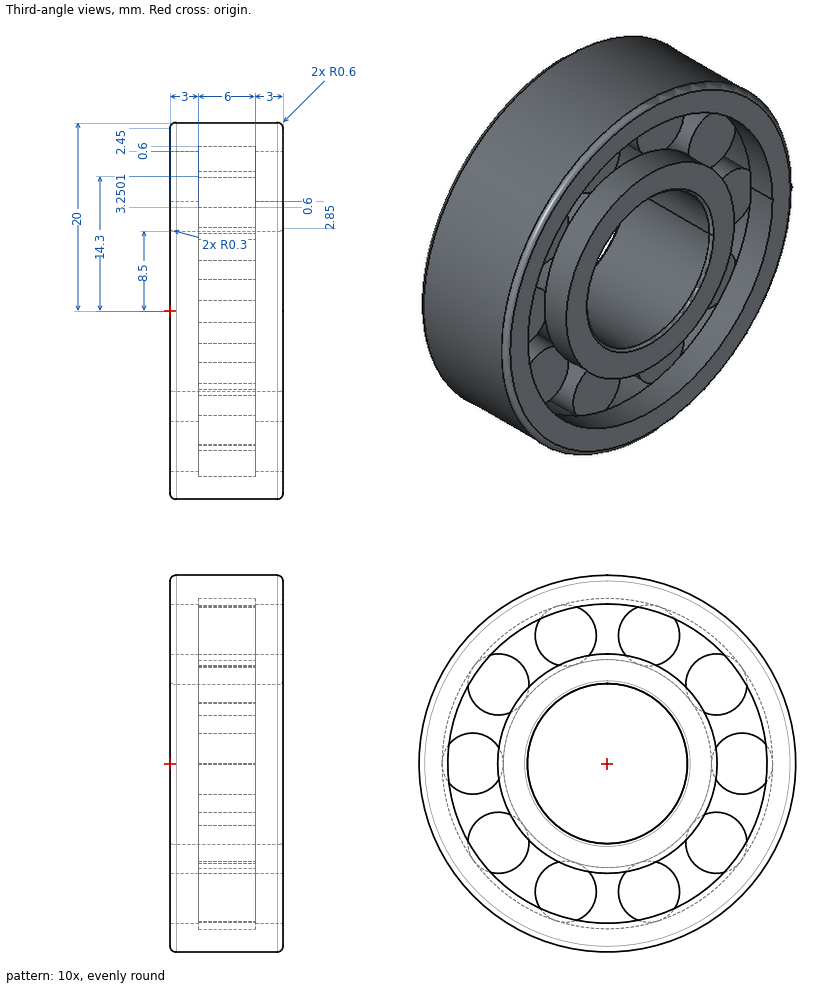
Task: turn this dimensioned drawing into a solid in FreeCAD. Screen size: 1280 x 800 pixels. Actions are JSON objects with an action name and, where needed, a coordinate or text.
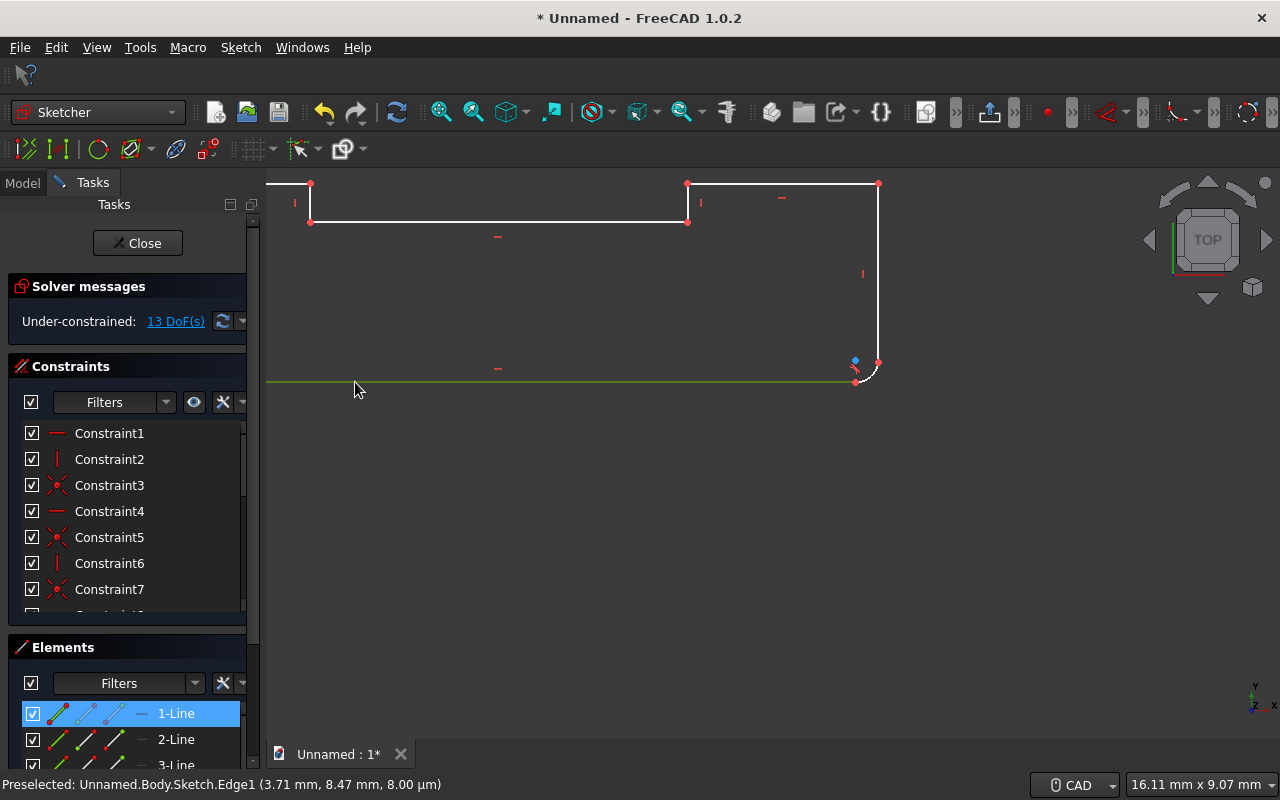
{"action": "scroll", "coordinate": [872, 376], "scroll_direction": "down", "scroll_amount": 4}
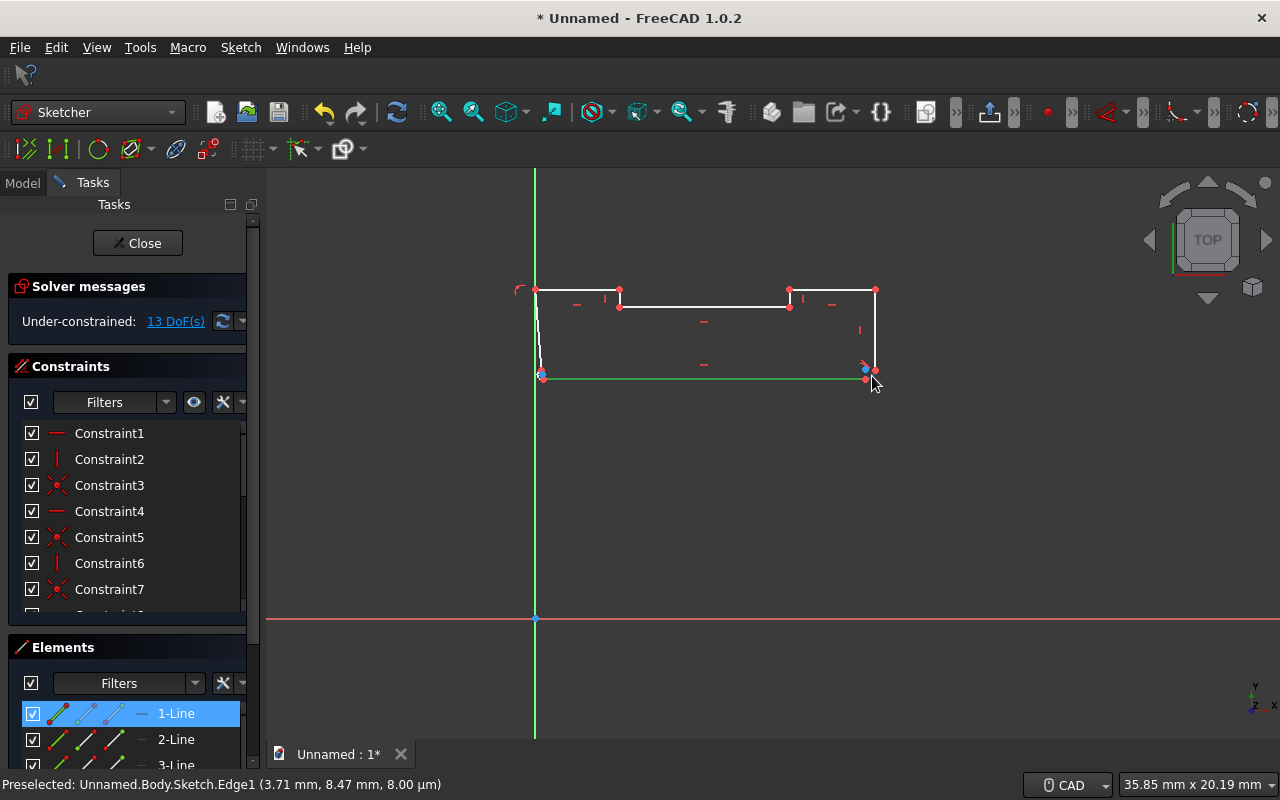
{"action": "scroll", "coordinate": [539, 378], "scroll_direction": "up", "scroll_amount": 7}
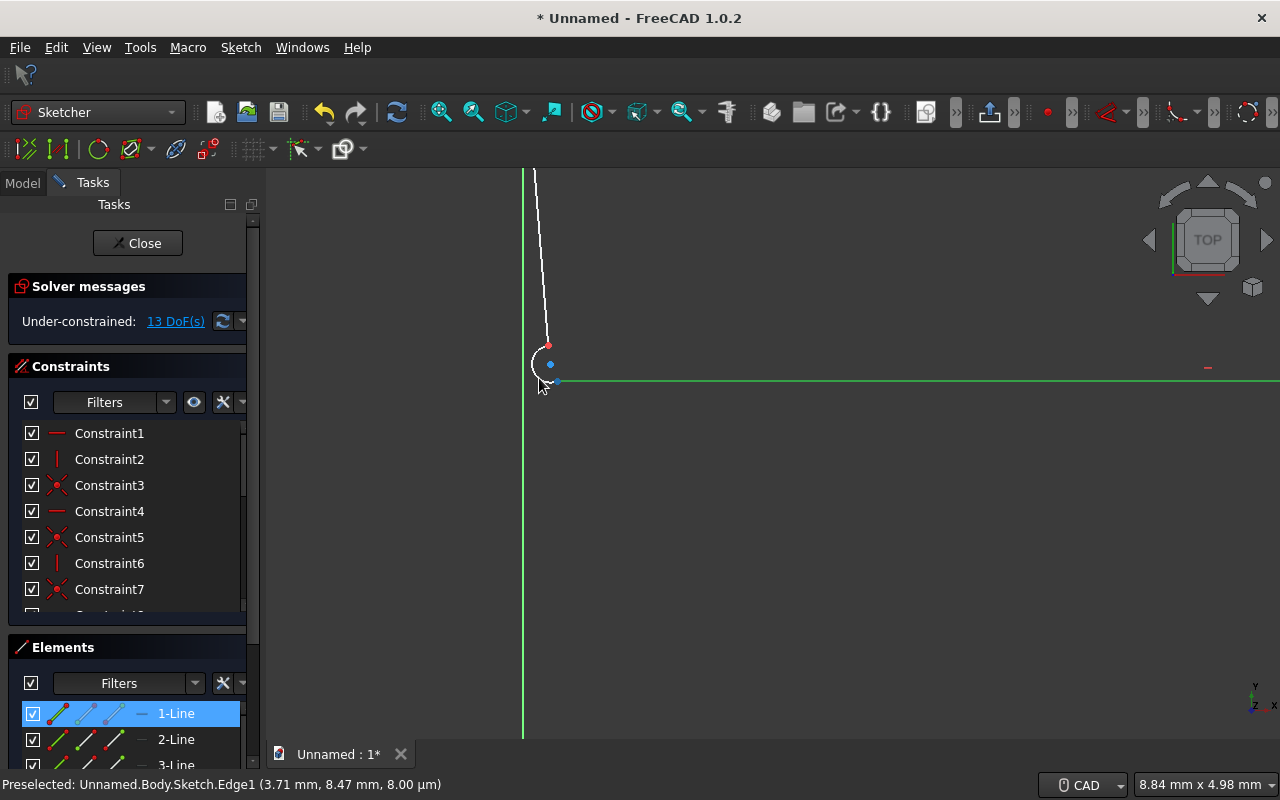
{"action": "left_click", "coordinate": [539, 379]}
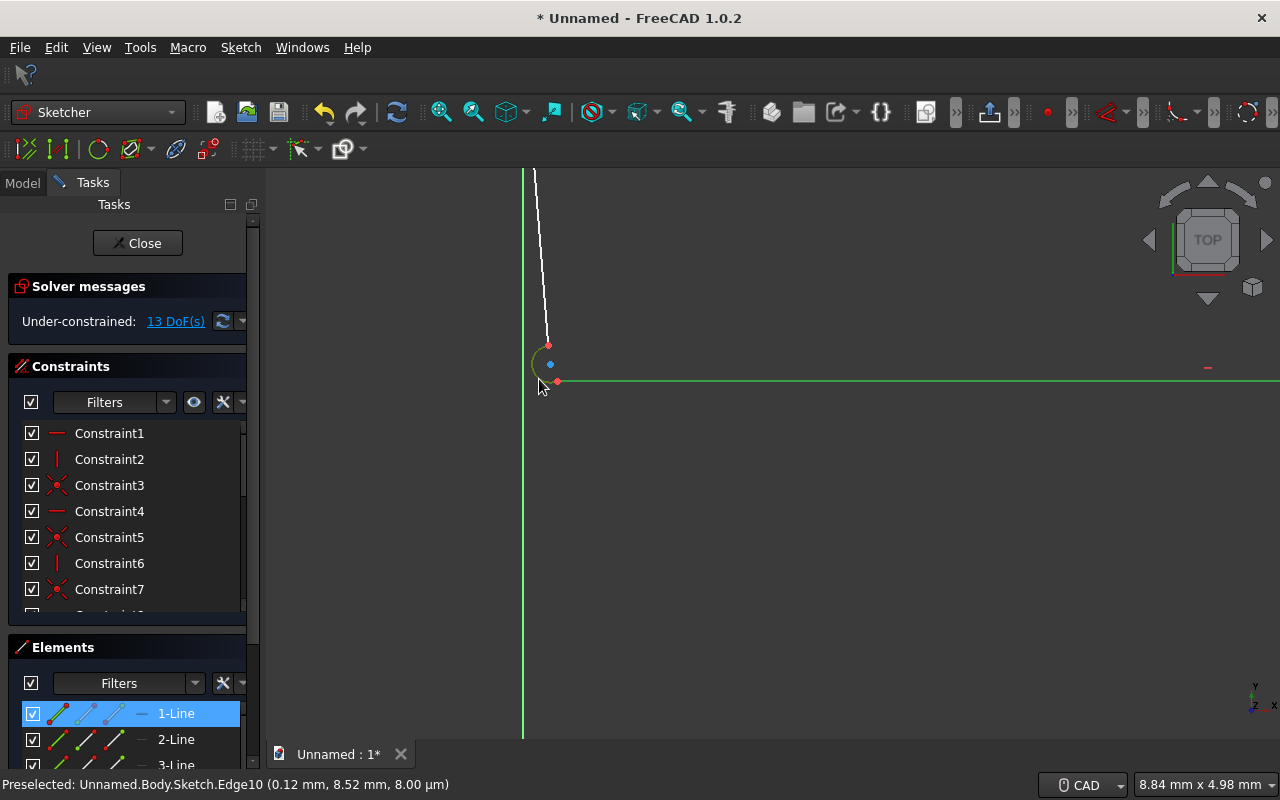
{"action": "key", "text": "t"}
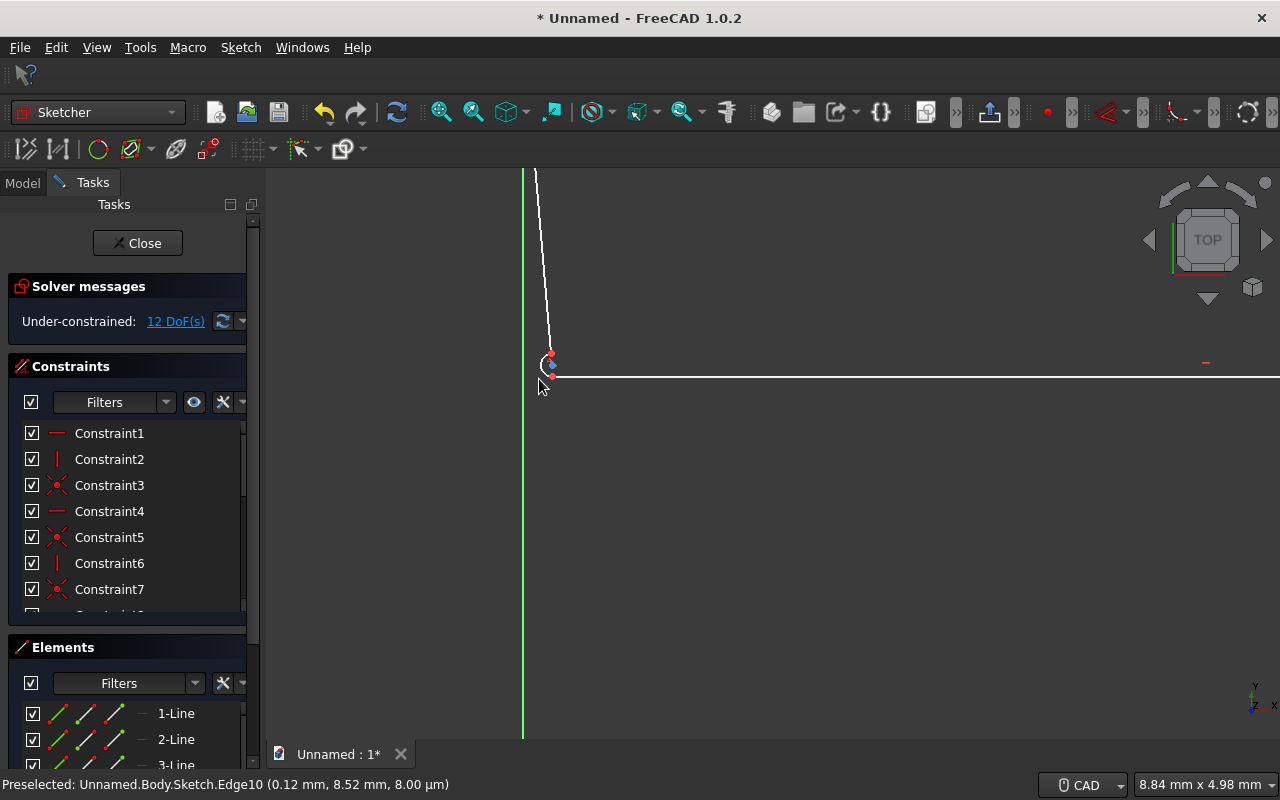
{"action": "scroll", "coordinate": [539, 378], "scroll_direction": "down", "scroll_amount": 7}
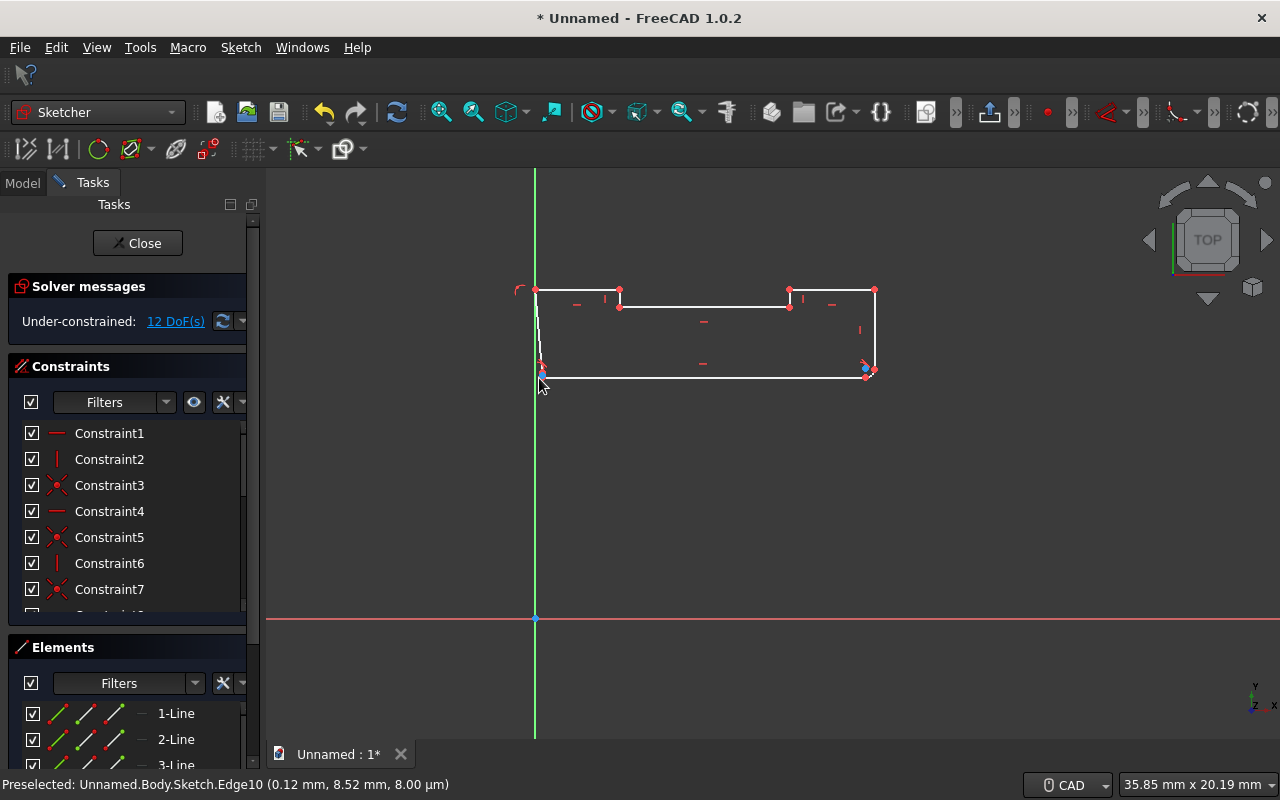
{"action": "left_click", "coordinate": [875, 346]}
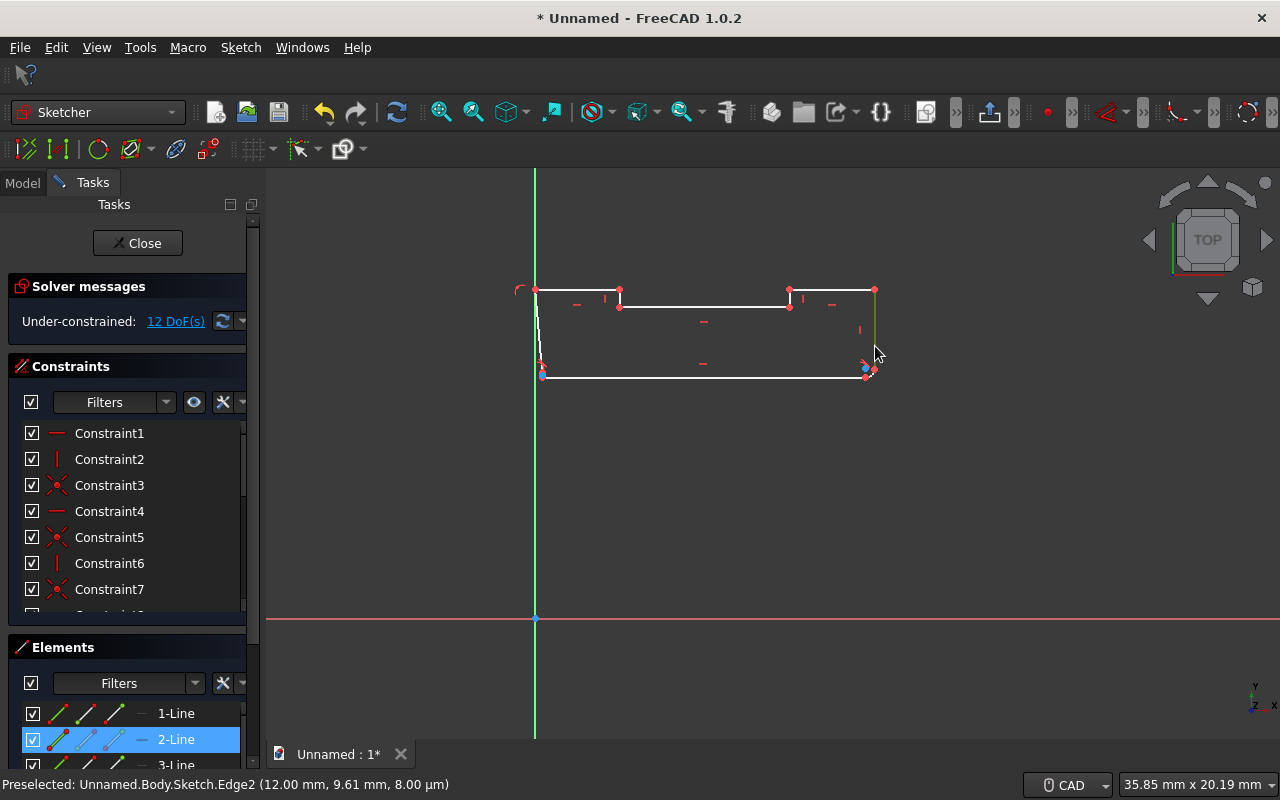
{"action": "scroll", "coordinate": [872, 376], "scroll_direction": "up", "scroll_amount": 4}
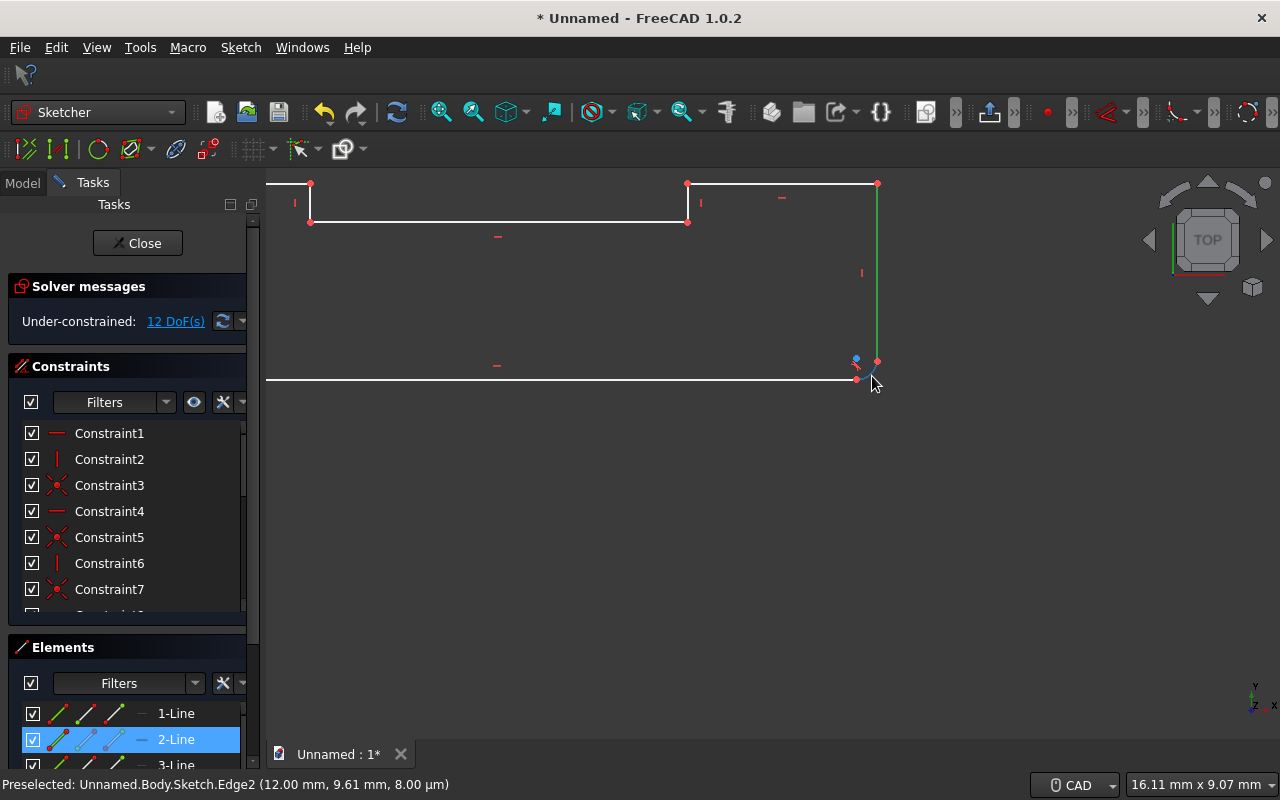
{"action": "left_click", "coordinate": [870, 375]}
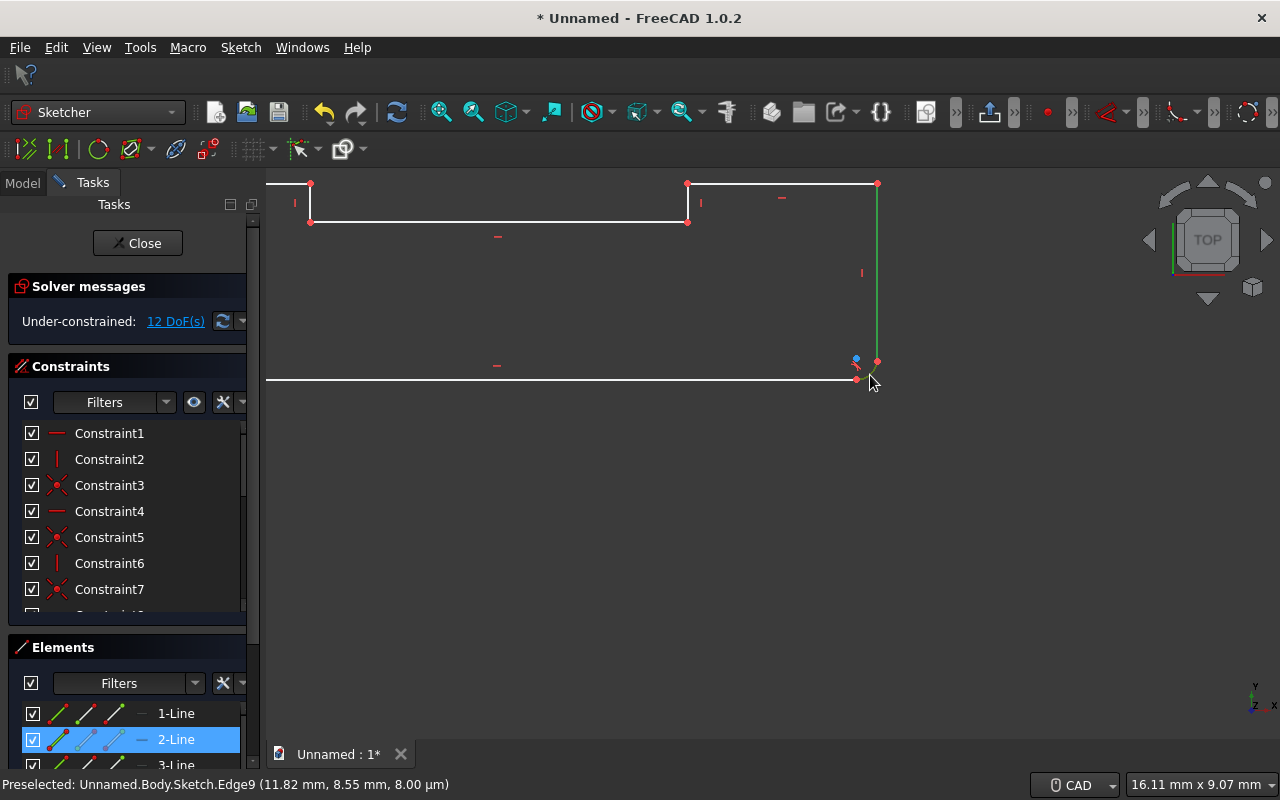
{"action": "key", "text": "t"}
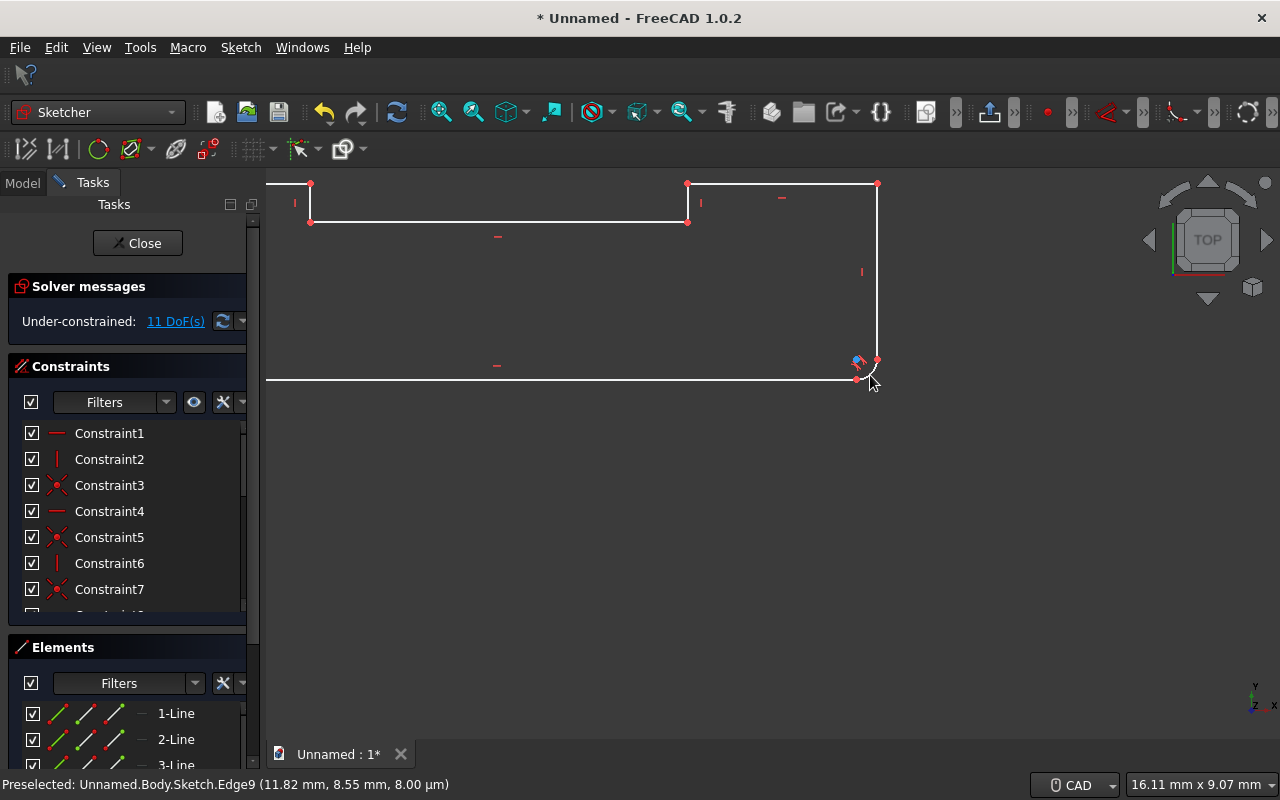
{"action": "scroll", "coordinate": [872, 376], "scroll_direction": "down", "scroll_amount": 4}